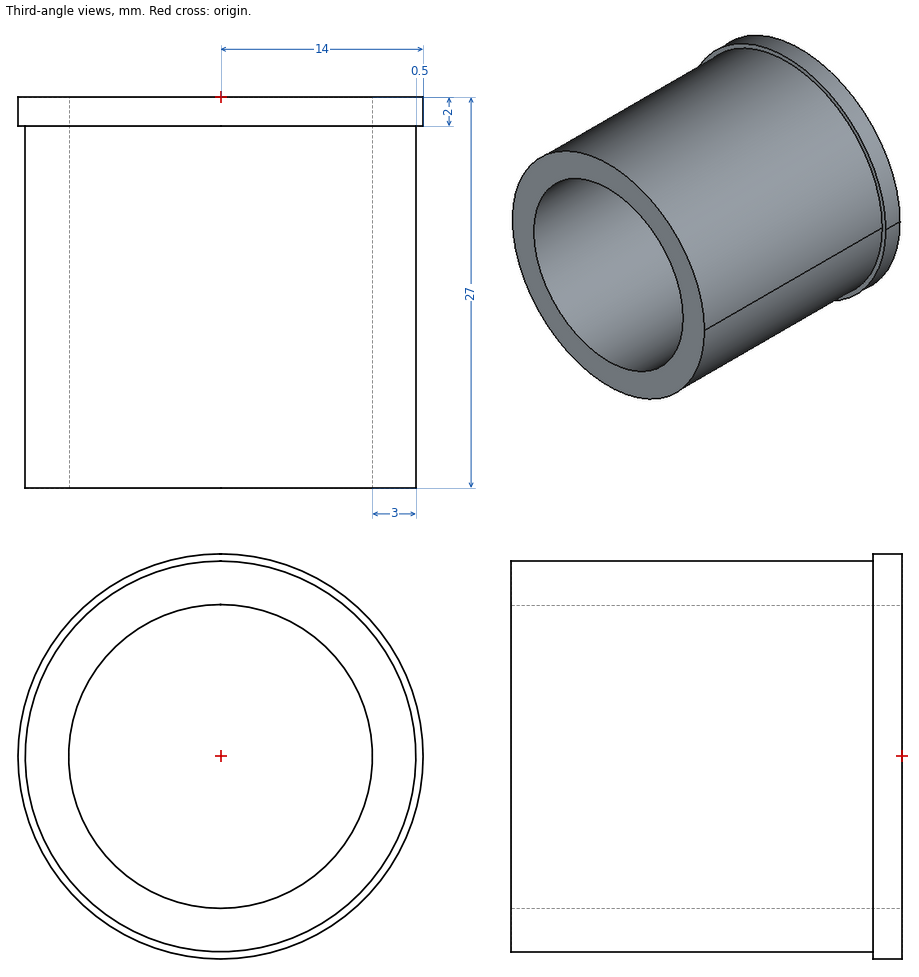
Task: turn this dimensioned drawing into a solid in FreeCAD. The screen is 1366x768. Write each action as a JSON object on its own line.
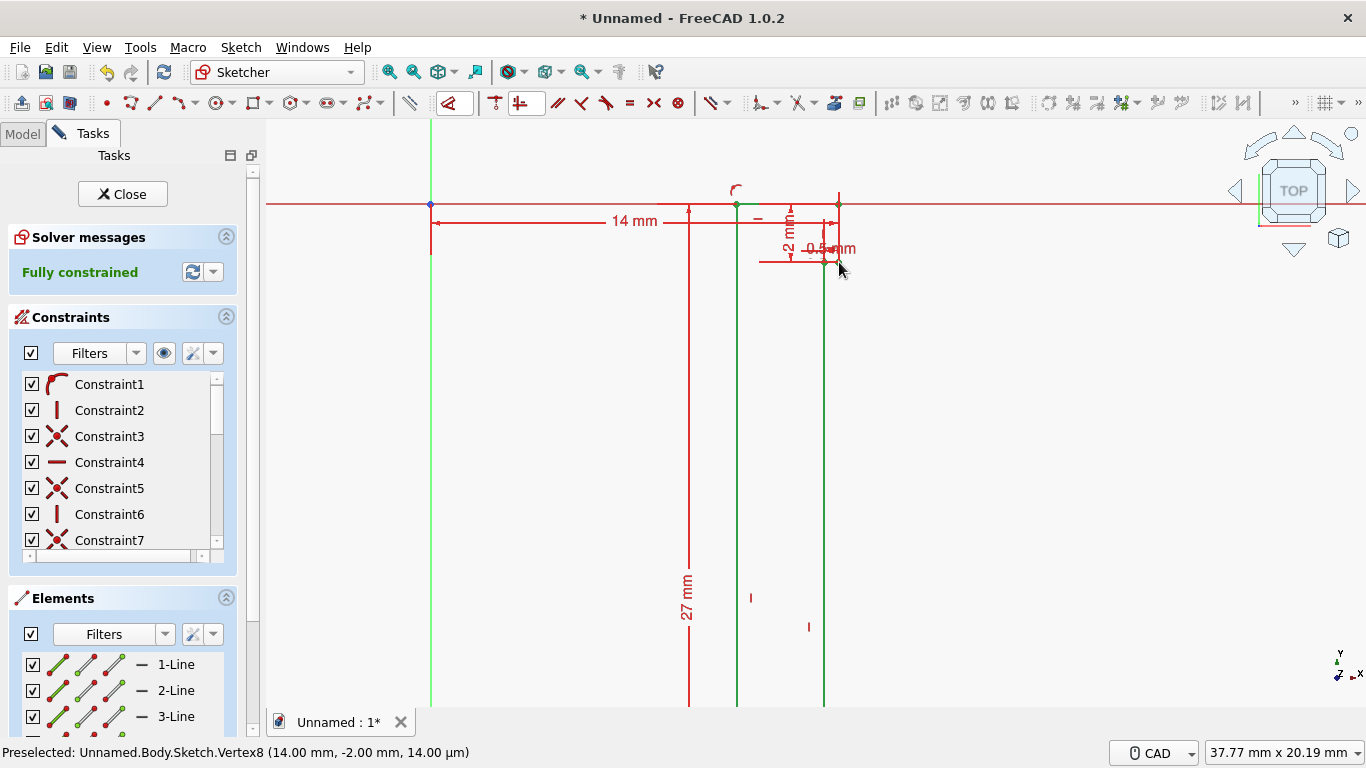
{"action": "left_click", "coordinate": [123, 194]}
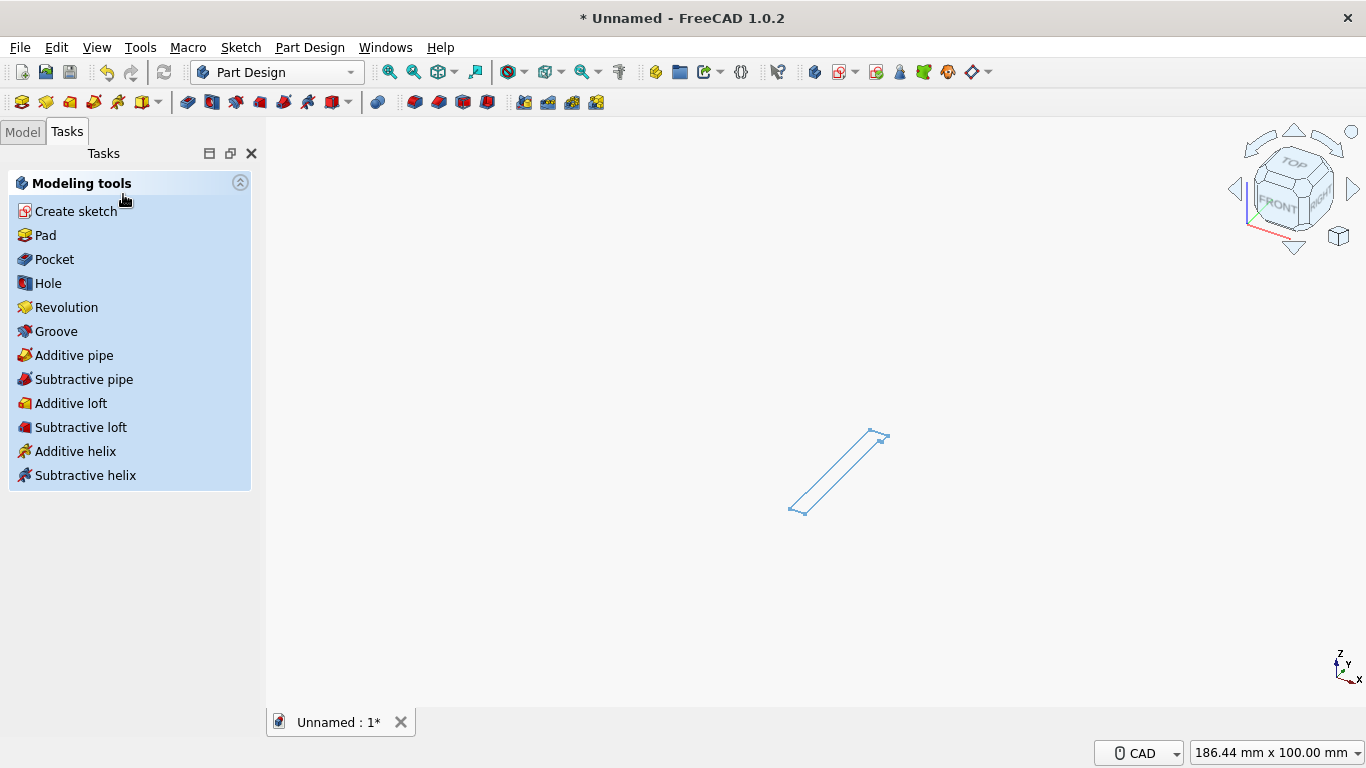
{"action": "left_click", "coordinate": [46, 102]}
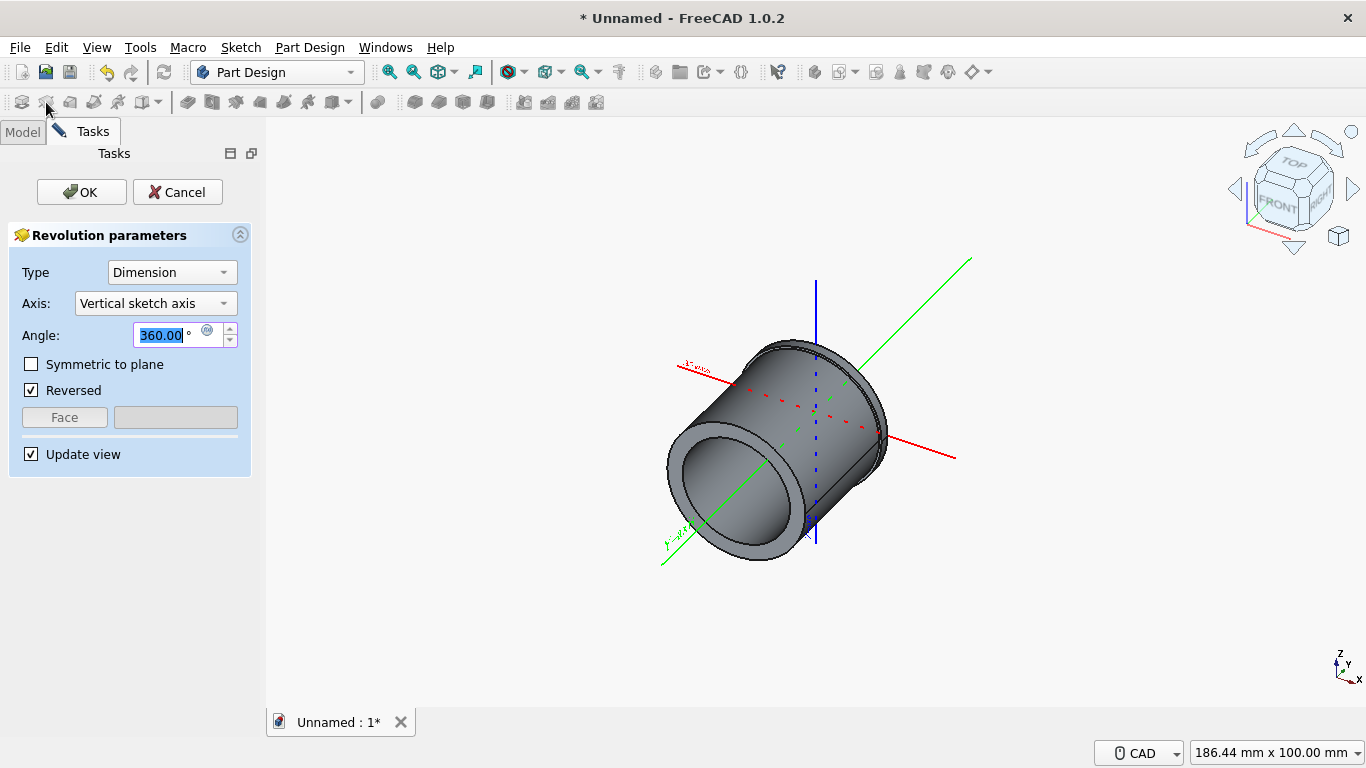
{"action": "left_click", "coordinate": [82, 192]}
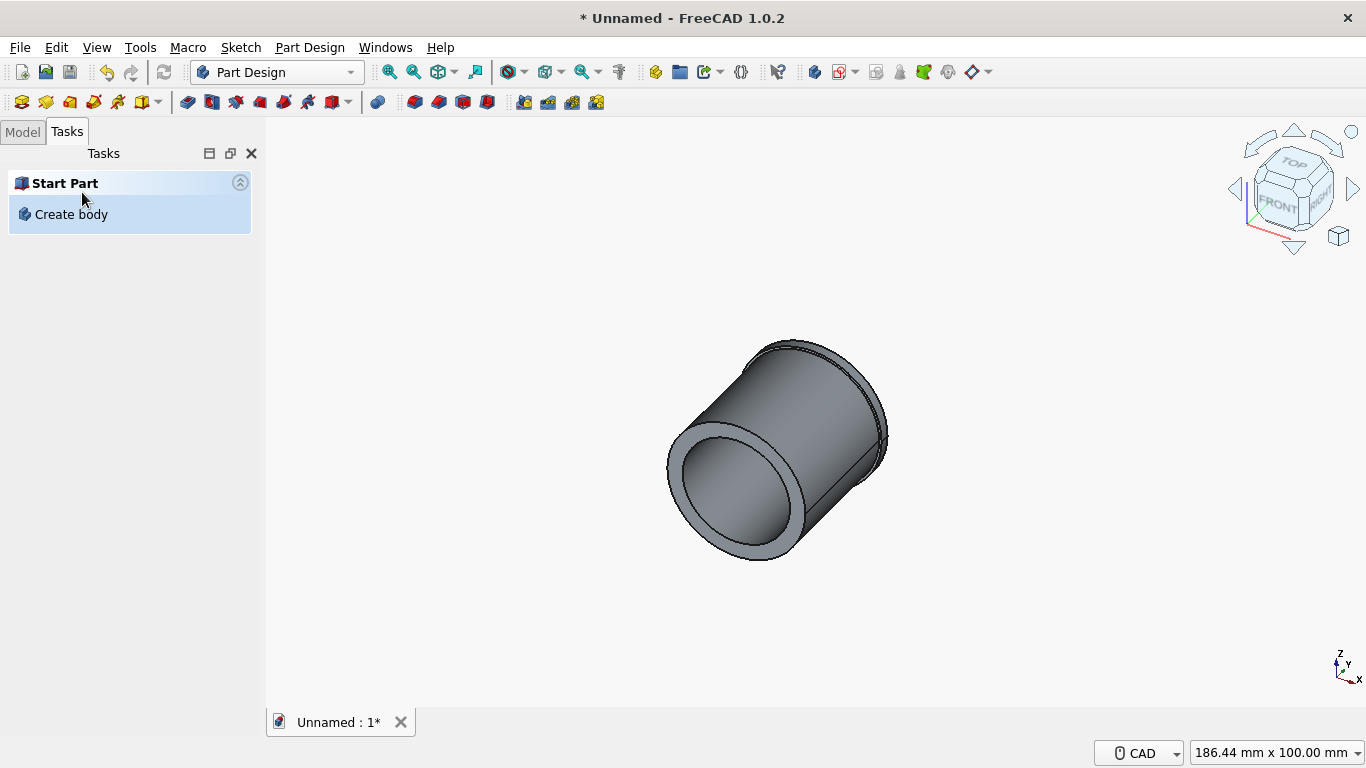
{"action": "key", "text": "0"}